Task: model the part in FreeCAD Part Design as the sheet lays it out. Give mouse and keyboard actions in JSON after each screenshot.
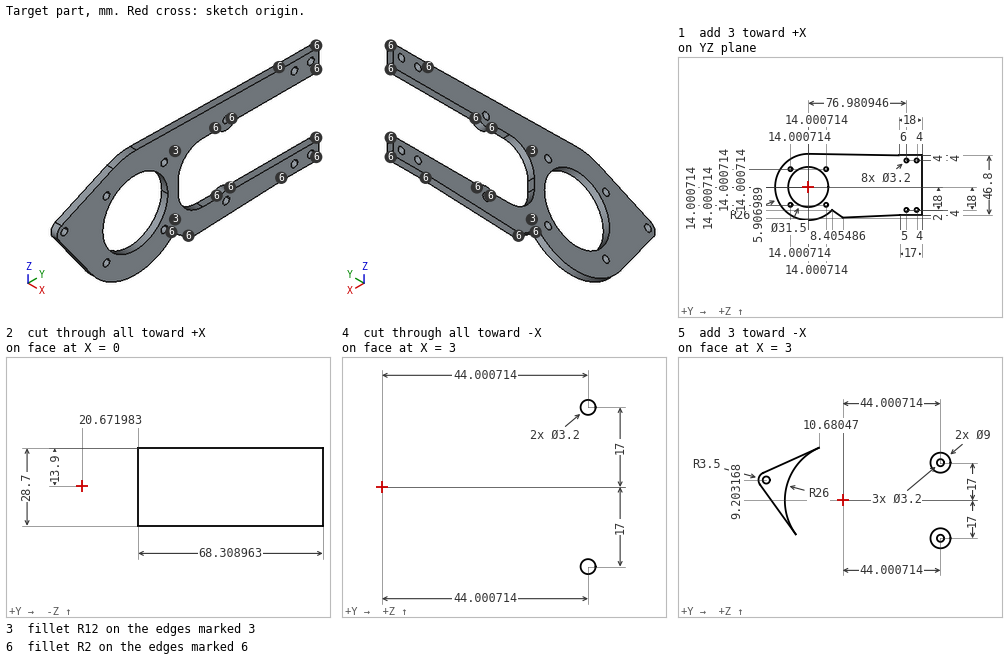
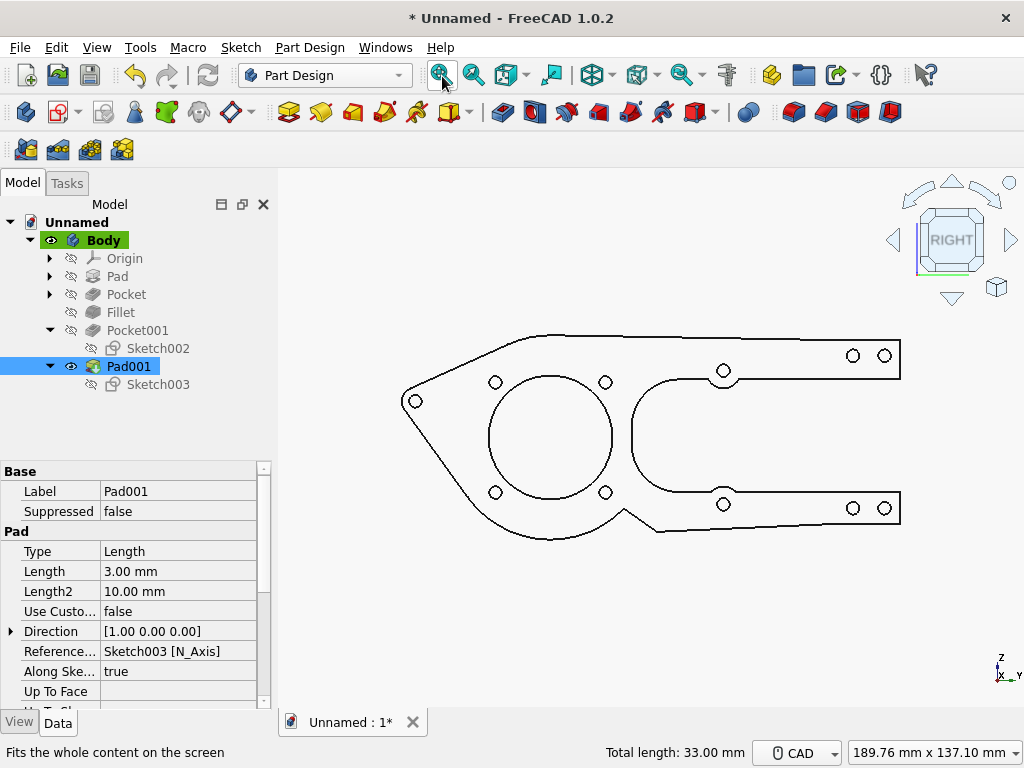
{"action": "key", "text": "5"}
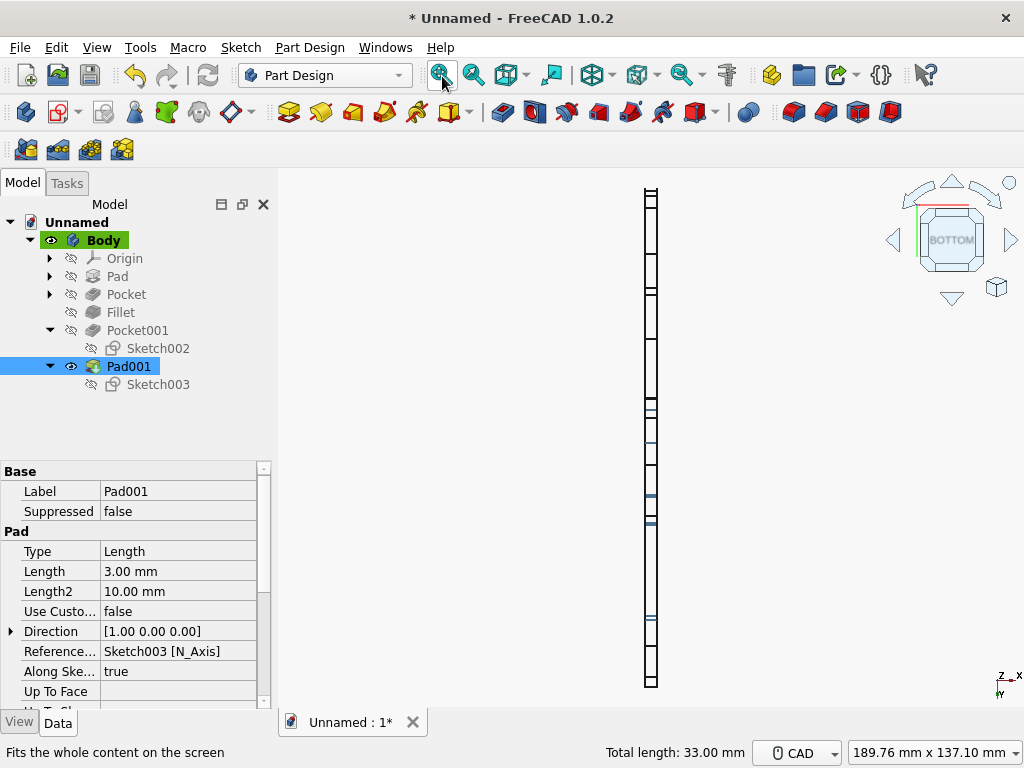
{"action": "key", "text": "4"}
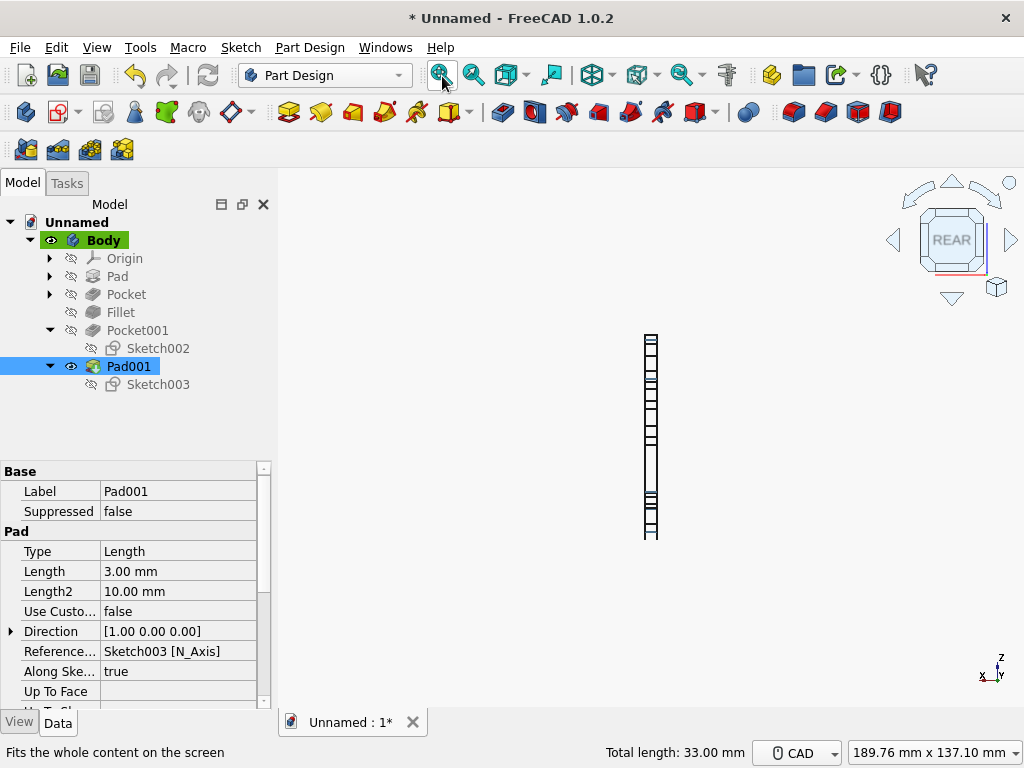
{"action": "left_click", "coordinate": [442, 76]}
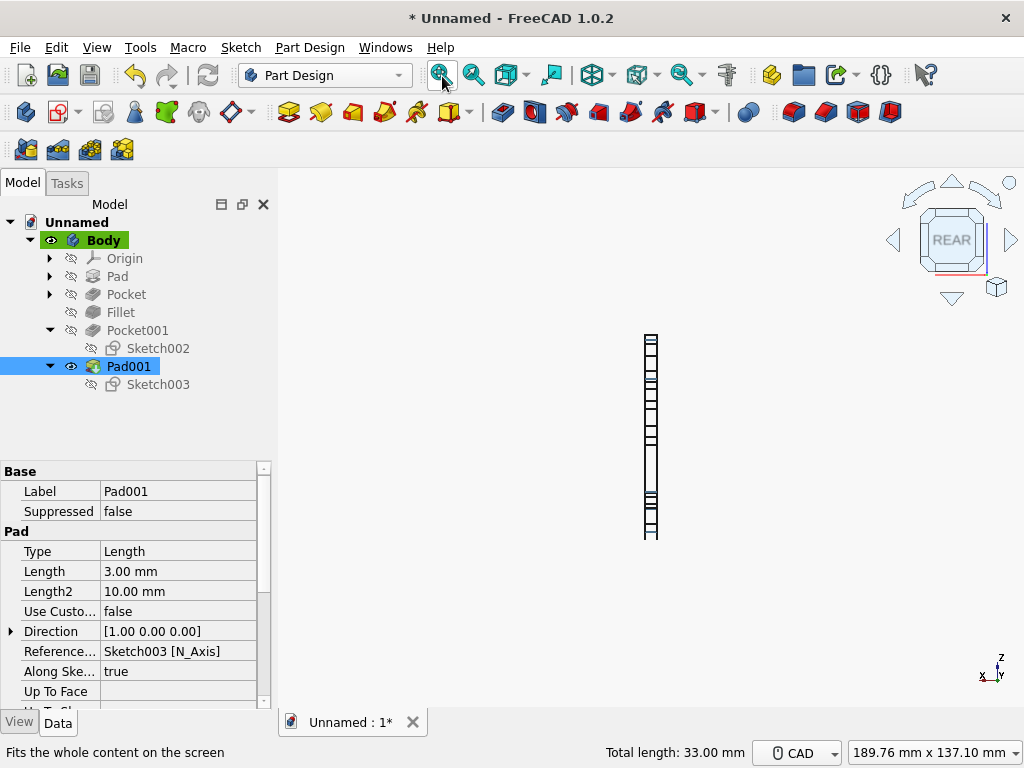
{"action": "scroll", "coordinate": [651, 523], "scroll_direction": "up", "scroll_amount": 7}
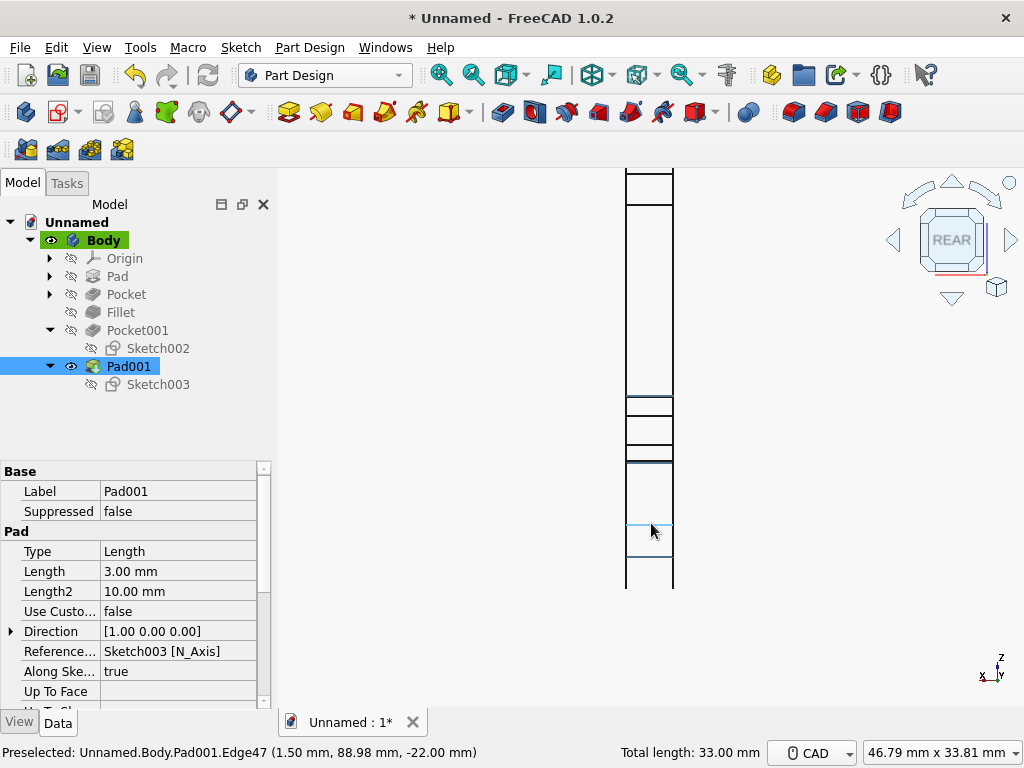
{"action": "left_click", "coordinate": [649, 524], "text": "ctrl"}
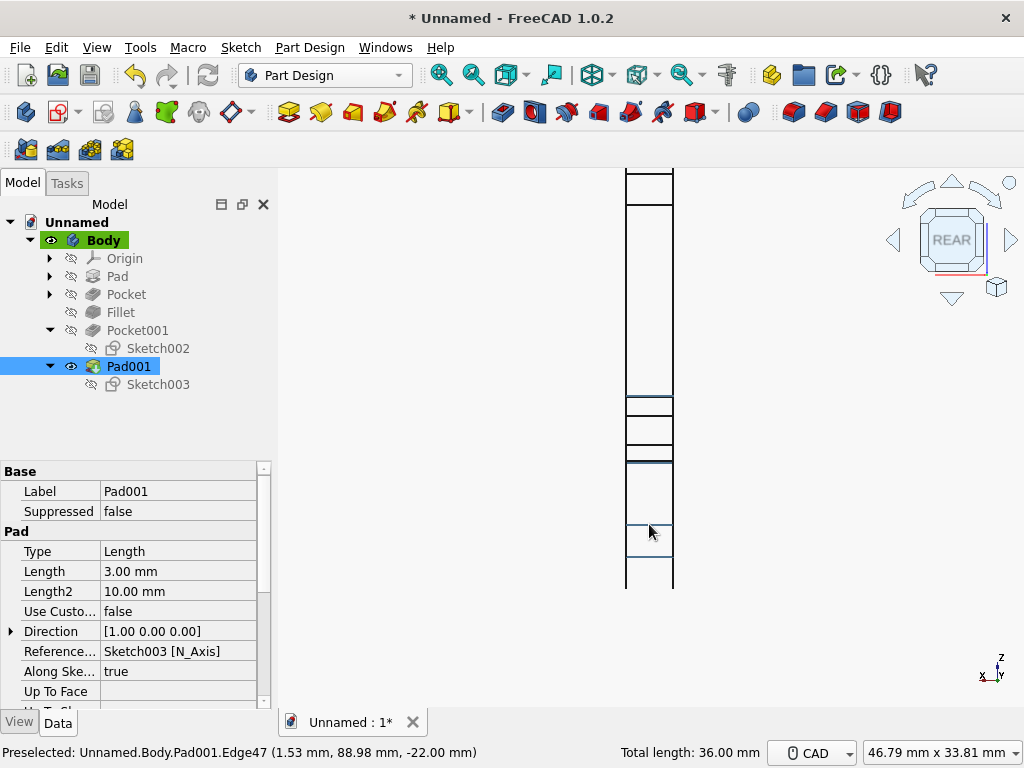
{"action": "key", "text": "v 1"}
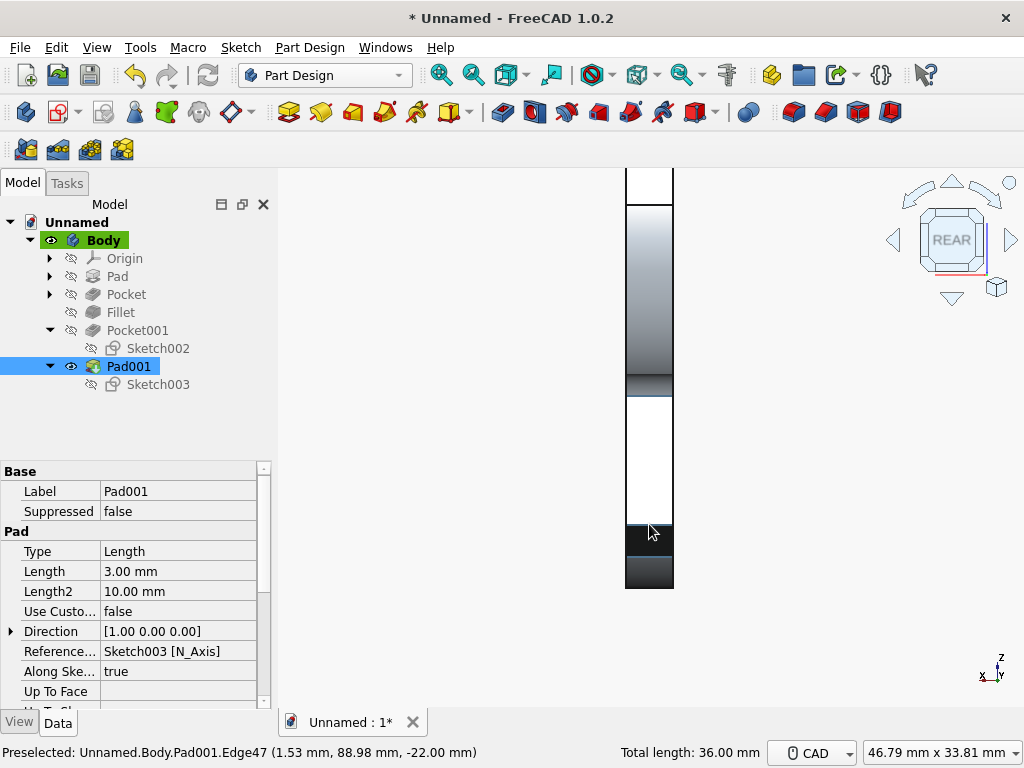
{"action": "left_click", "coordinate": [794, 112]}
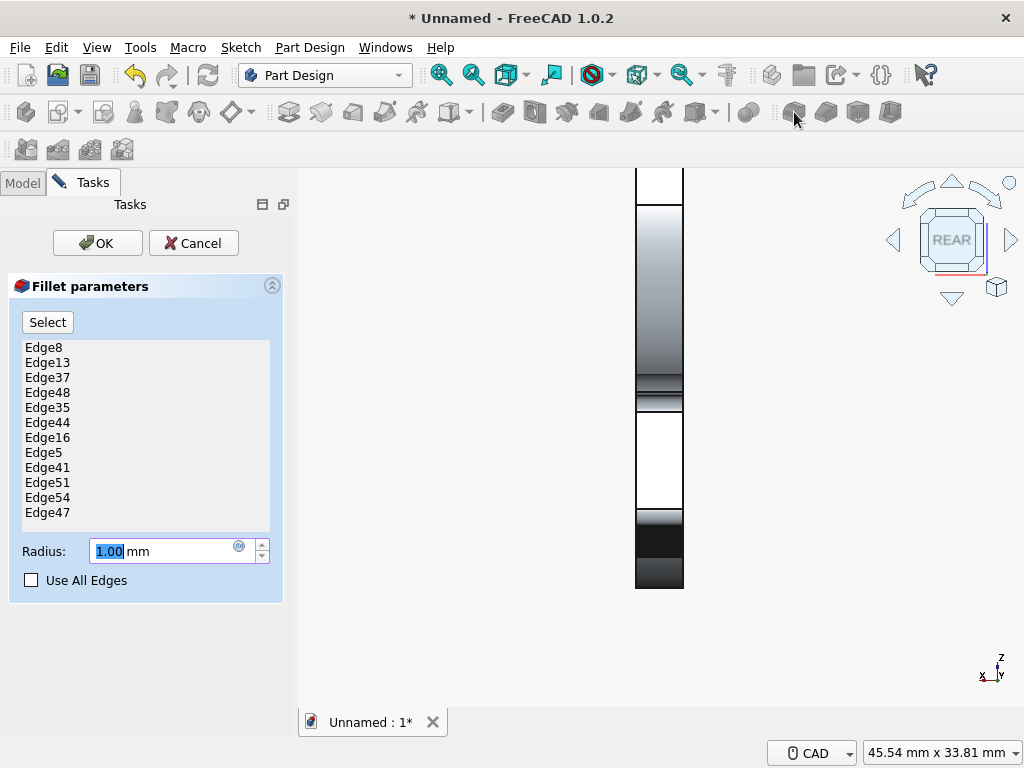
{"action": "type", "text": "2"}
{"action": "key", "text": "Tab"}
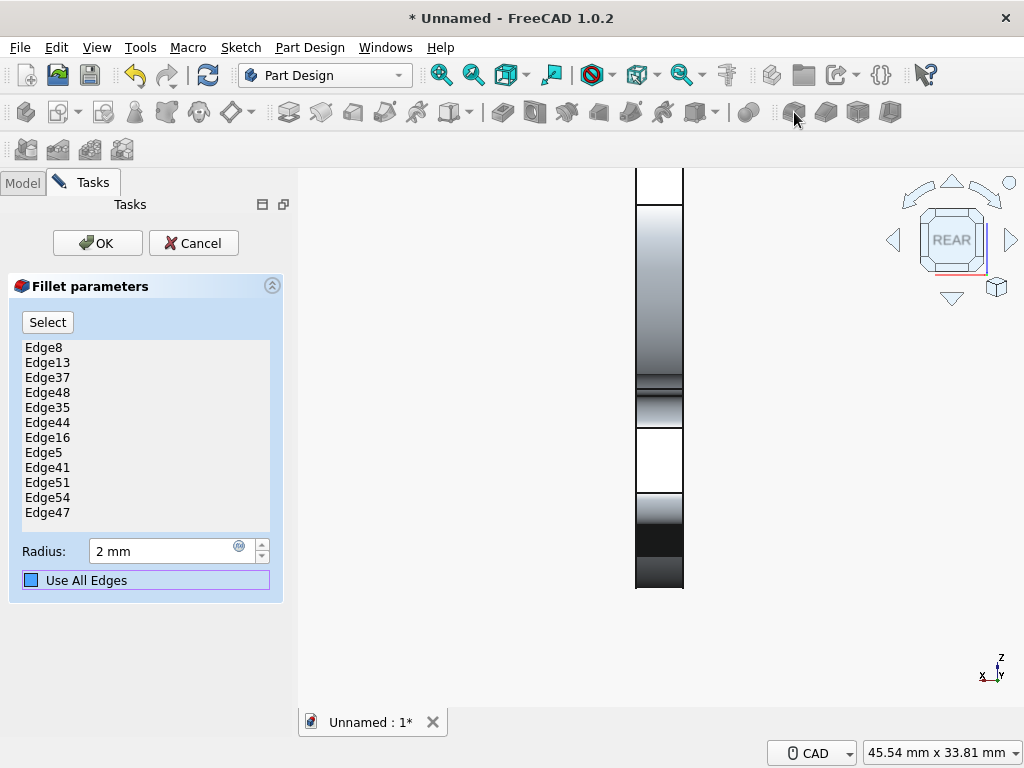
{"action": "left_click", "coordinate": [98, 243]}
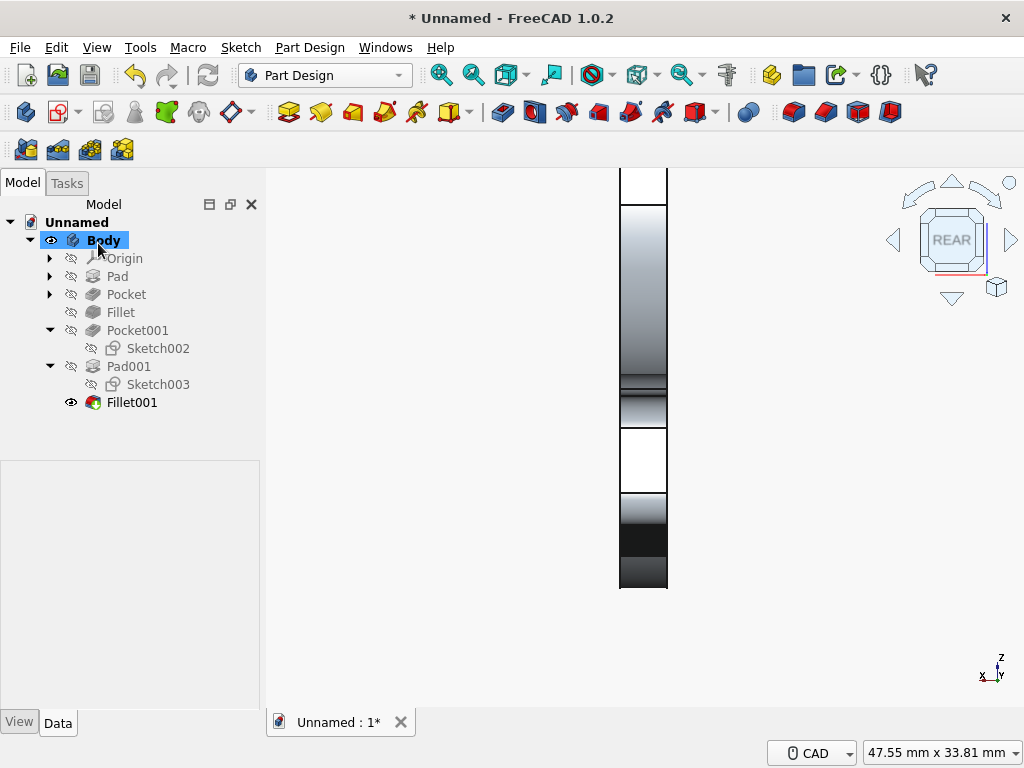
{"action": "key", "text": "0"}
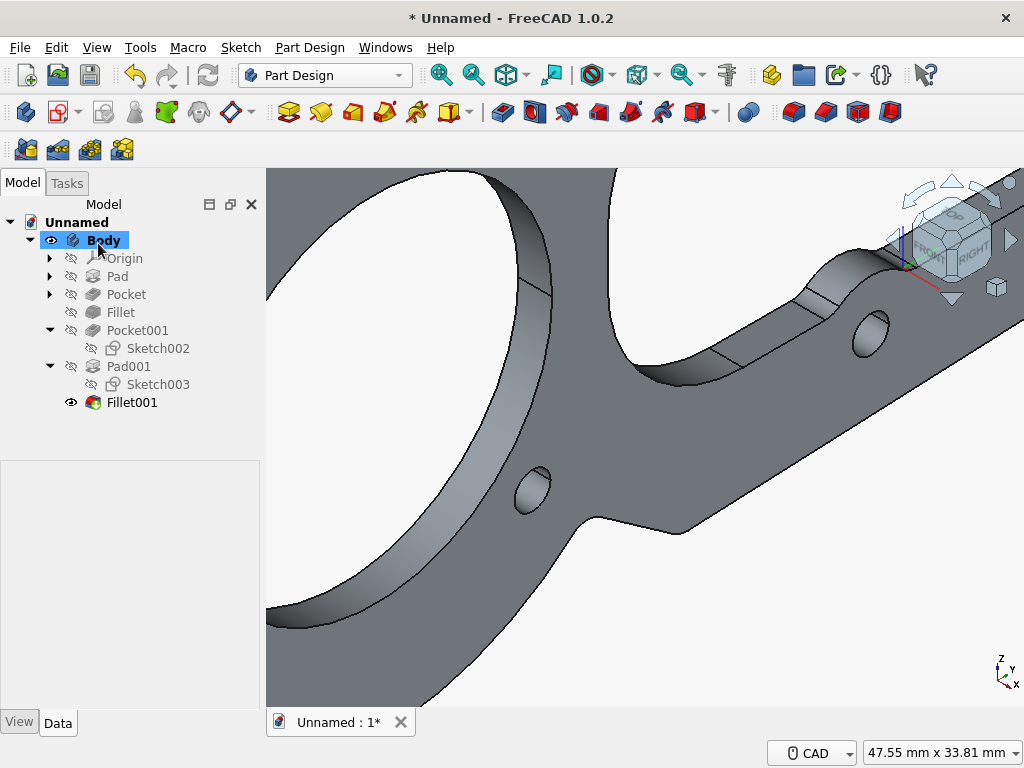
{"action": "left_click", "coordinate": [442, 76]}